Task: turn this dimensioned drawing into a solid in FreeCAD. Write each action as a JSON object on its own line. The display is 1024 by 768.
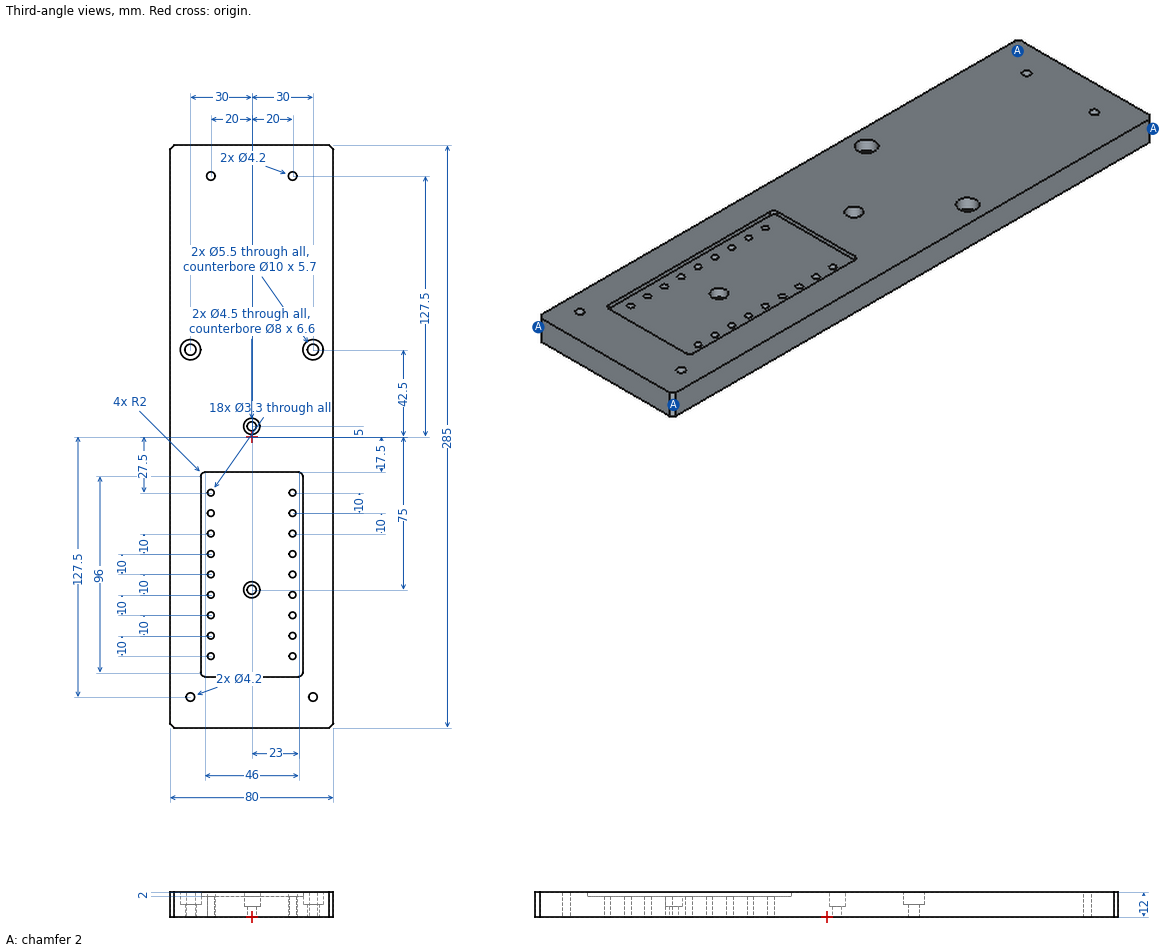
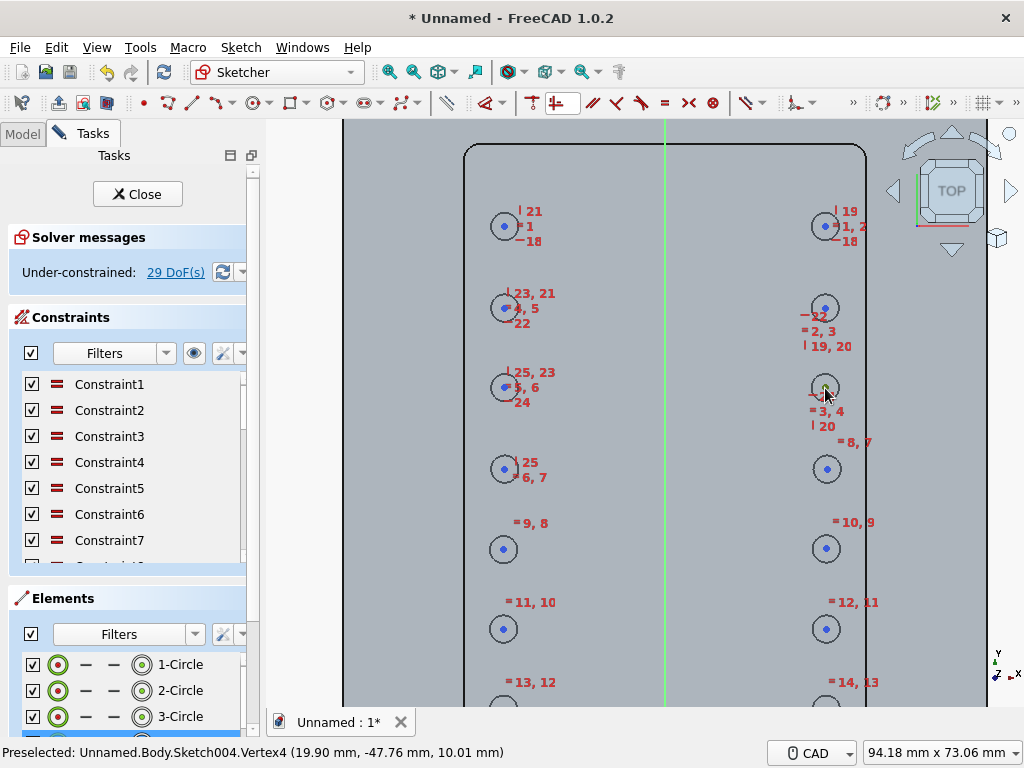
{"action": "left_click", "coordinate": [827, 469]}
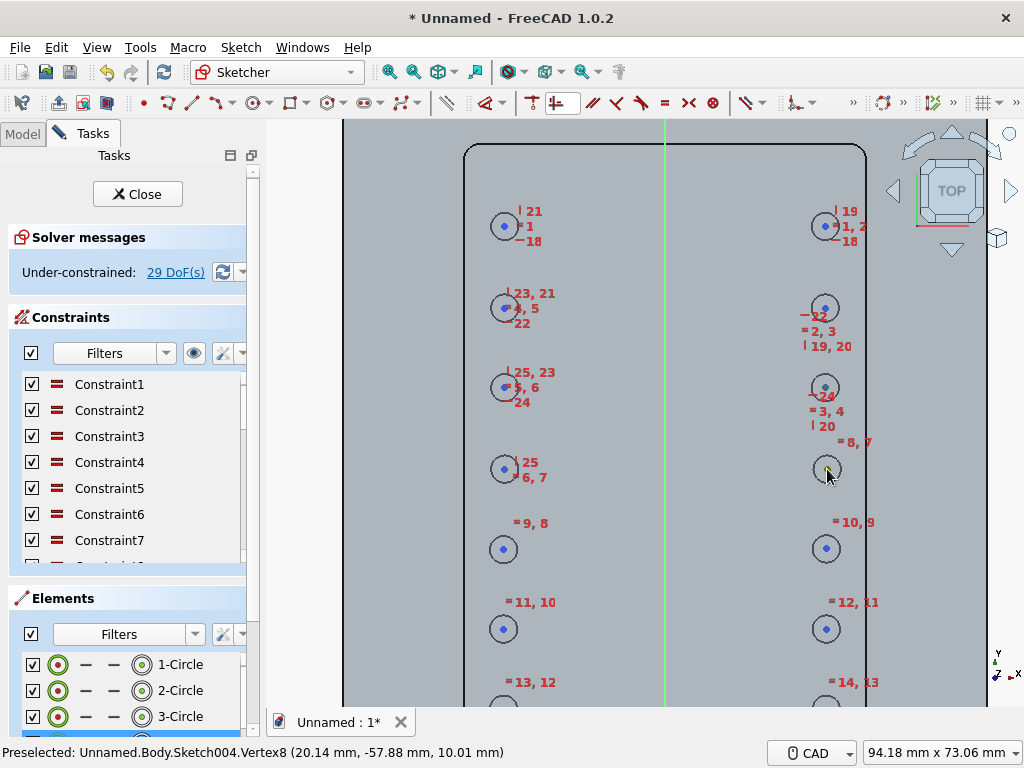
{"action": "key", "text": "v"}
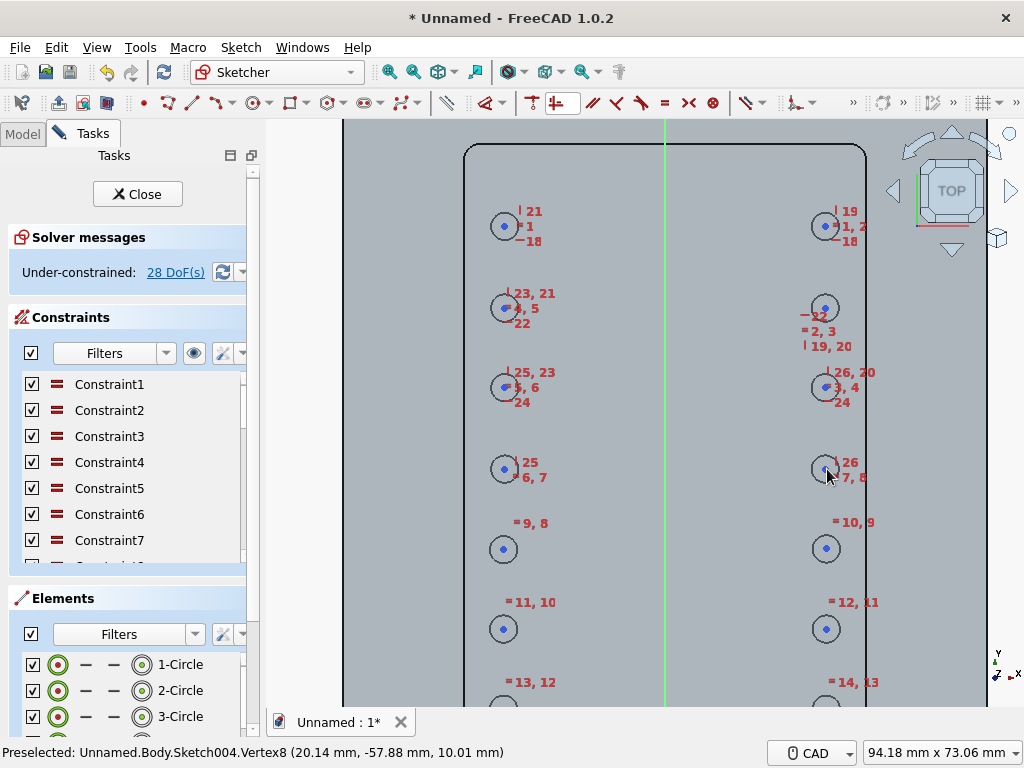
{"action": "left_click", "coordinate": [505, 469]}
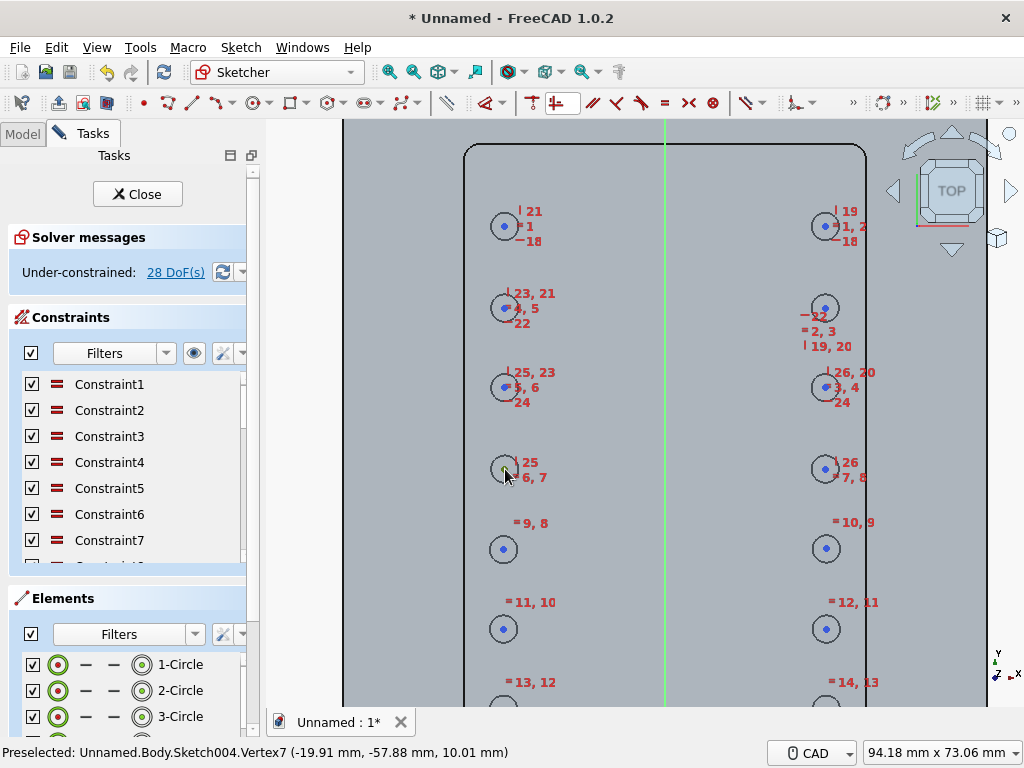
{"action": "left_click", "coordinate": [825, 469]}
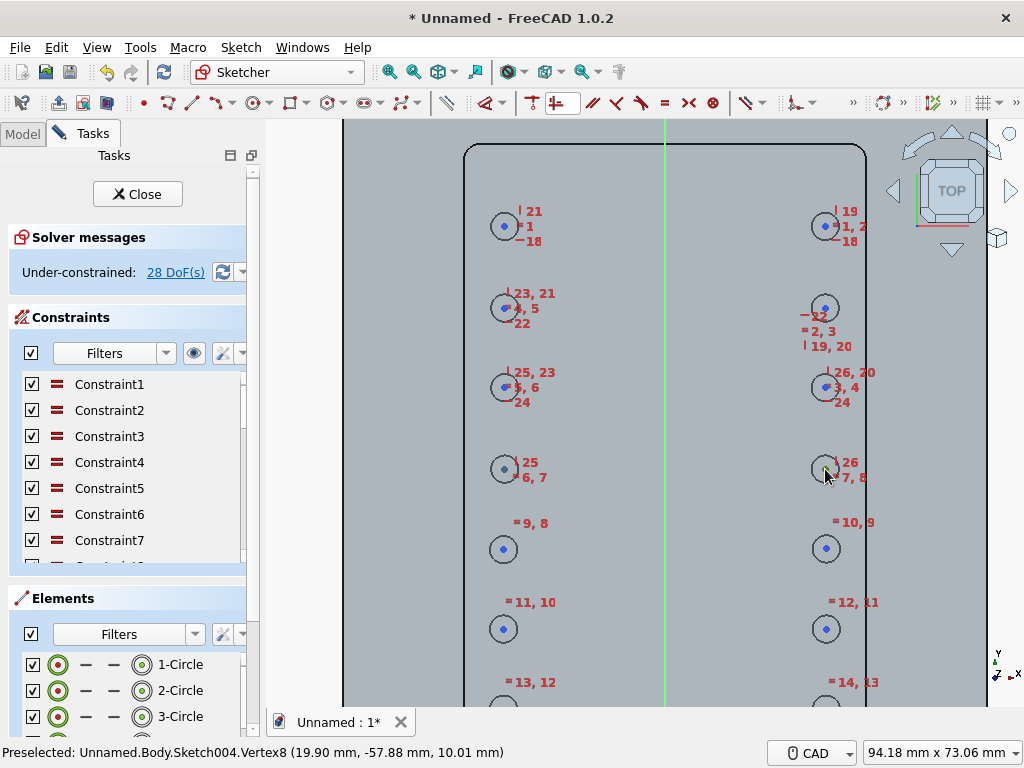
{"action": "key", "text": "h"}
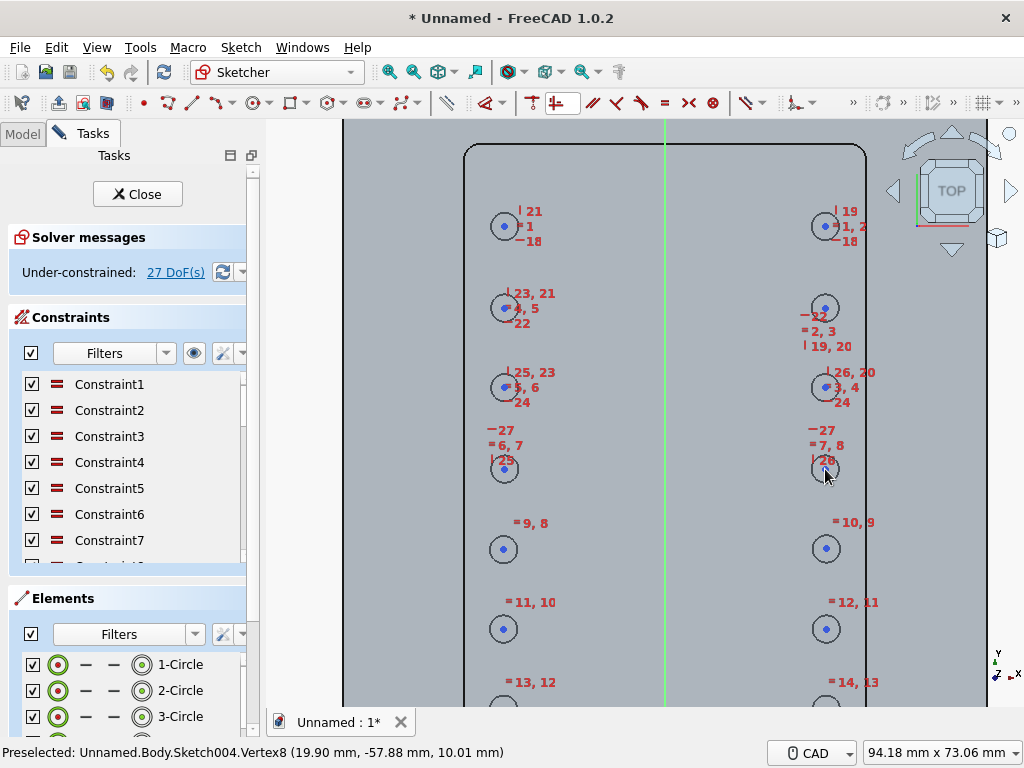
{"action": "left_click", "coordinate": [505, 469]}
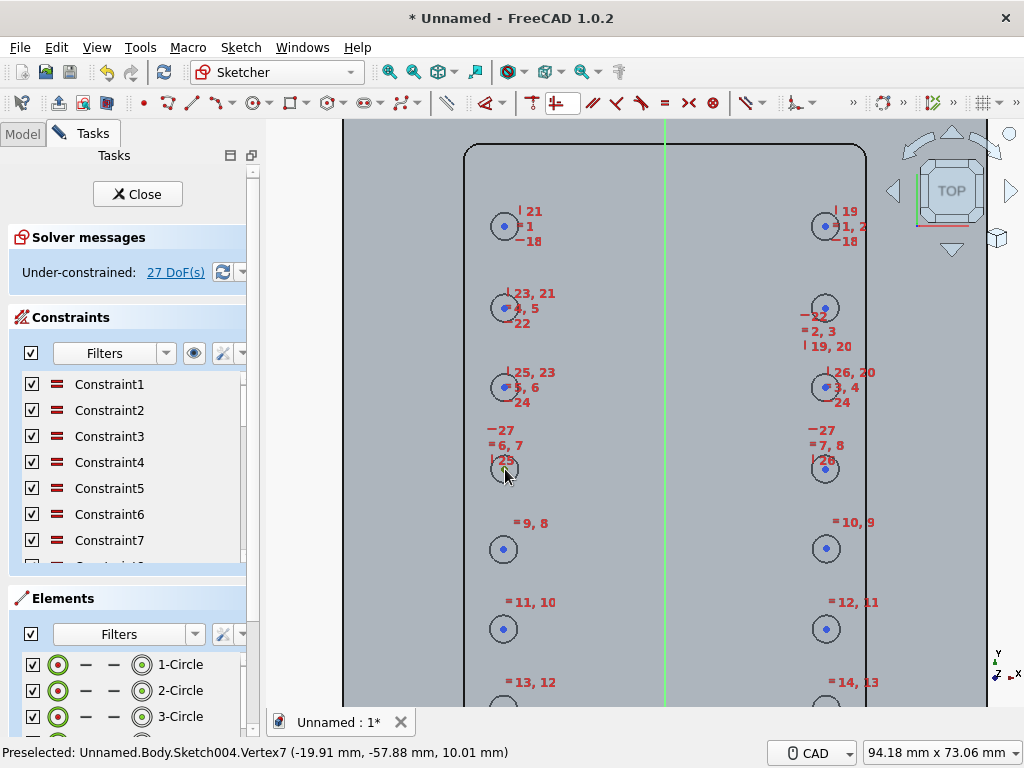
{"action": "left_click", "coordinate": [504, 550]}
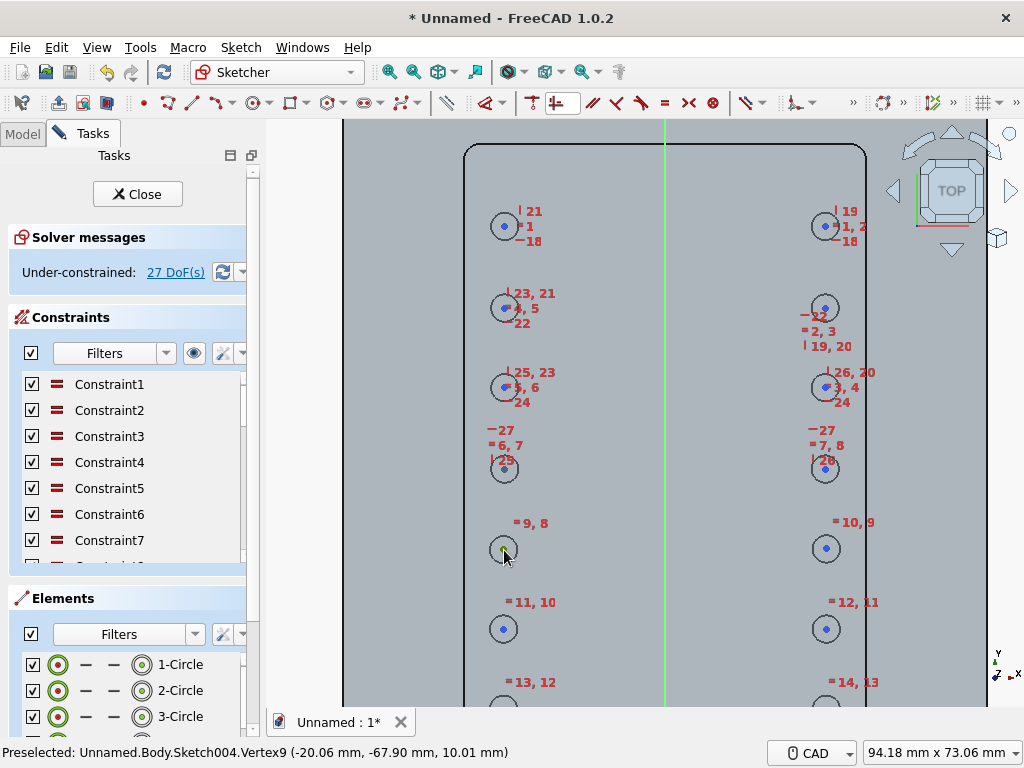
{"action": "key", "text": "v"}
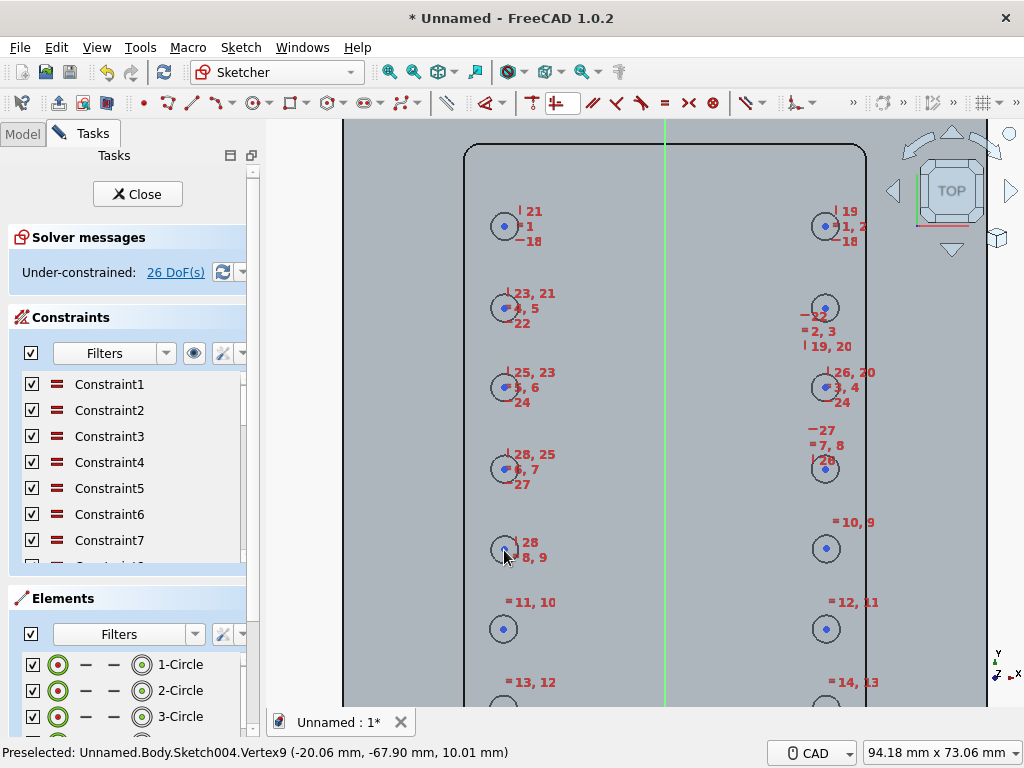
{"action": "left_click", "coordinate": [825, 469]}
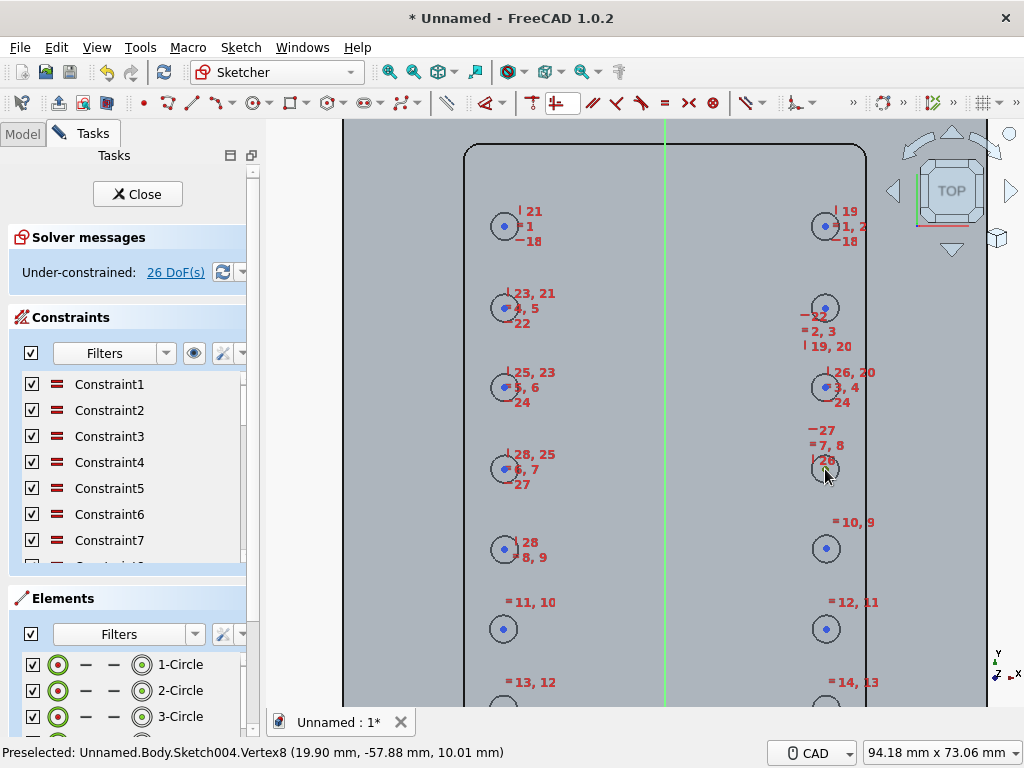
{"action": "left_click", "coordinate": [826, 549]}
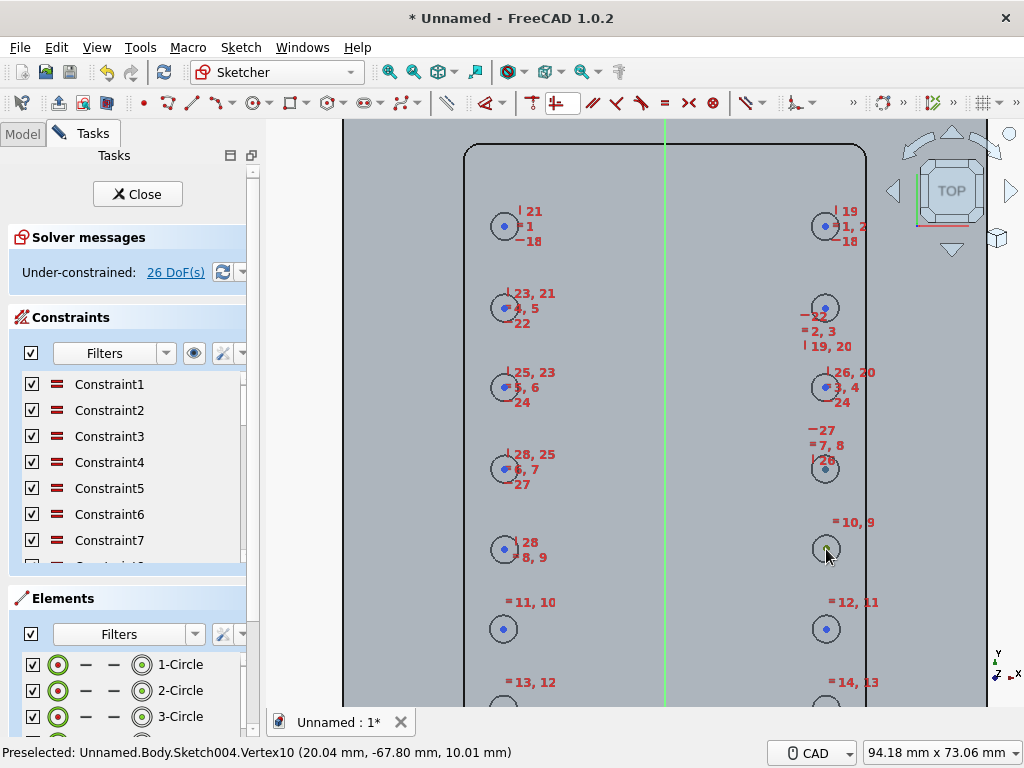
{"action": "key", "text": "v"}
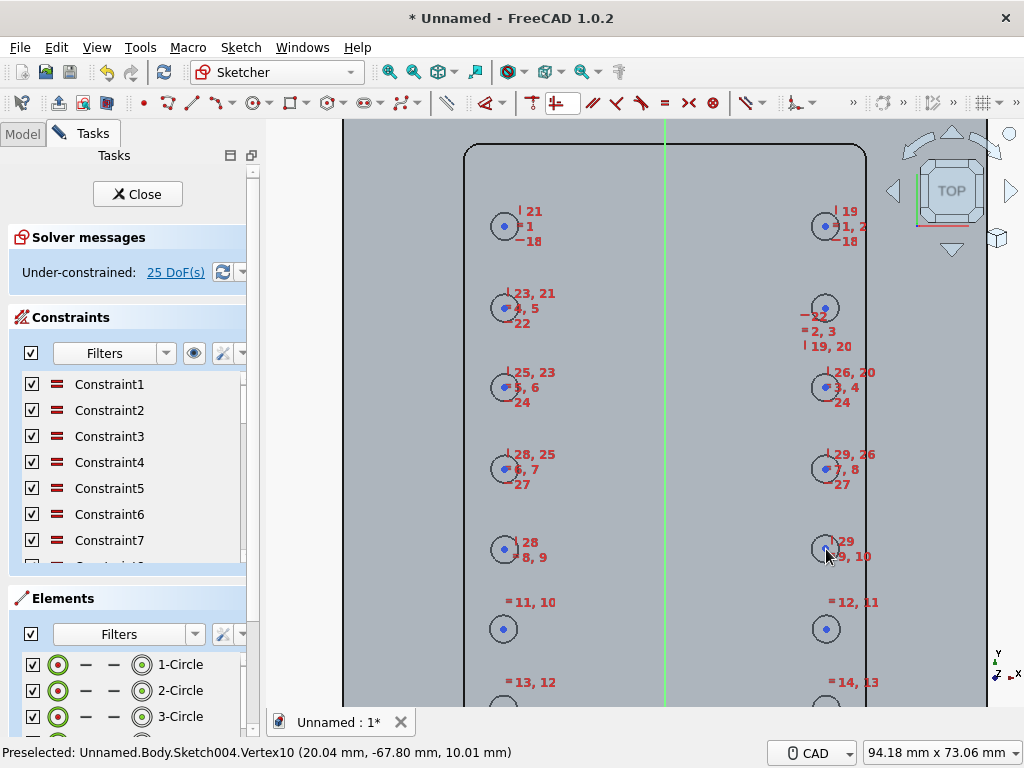
{"action": "left_click", "coordinate": [505, 550]}